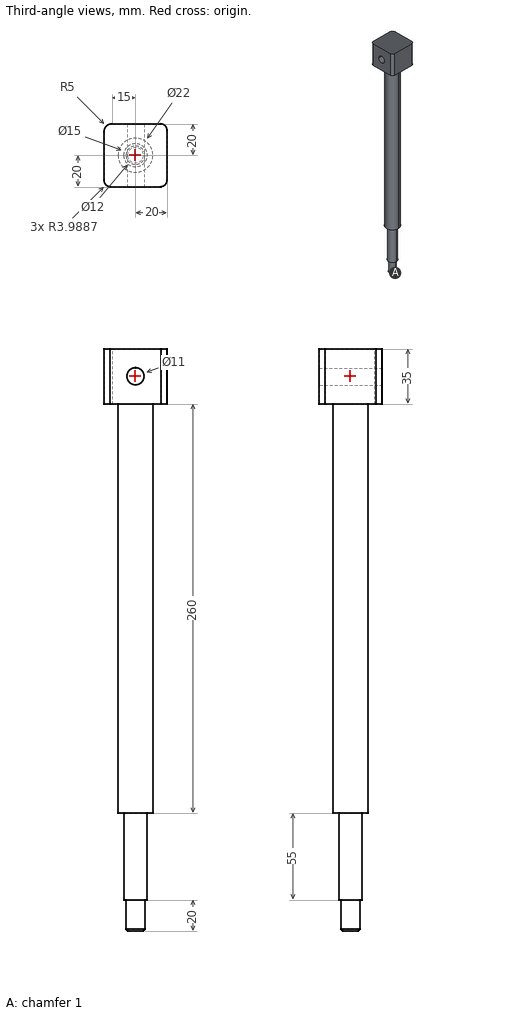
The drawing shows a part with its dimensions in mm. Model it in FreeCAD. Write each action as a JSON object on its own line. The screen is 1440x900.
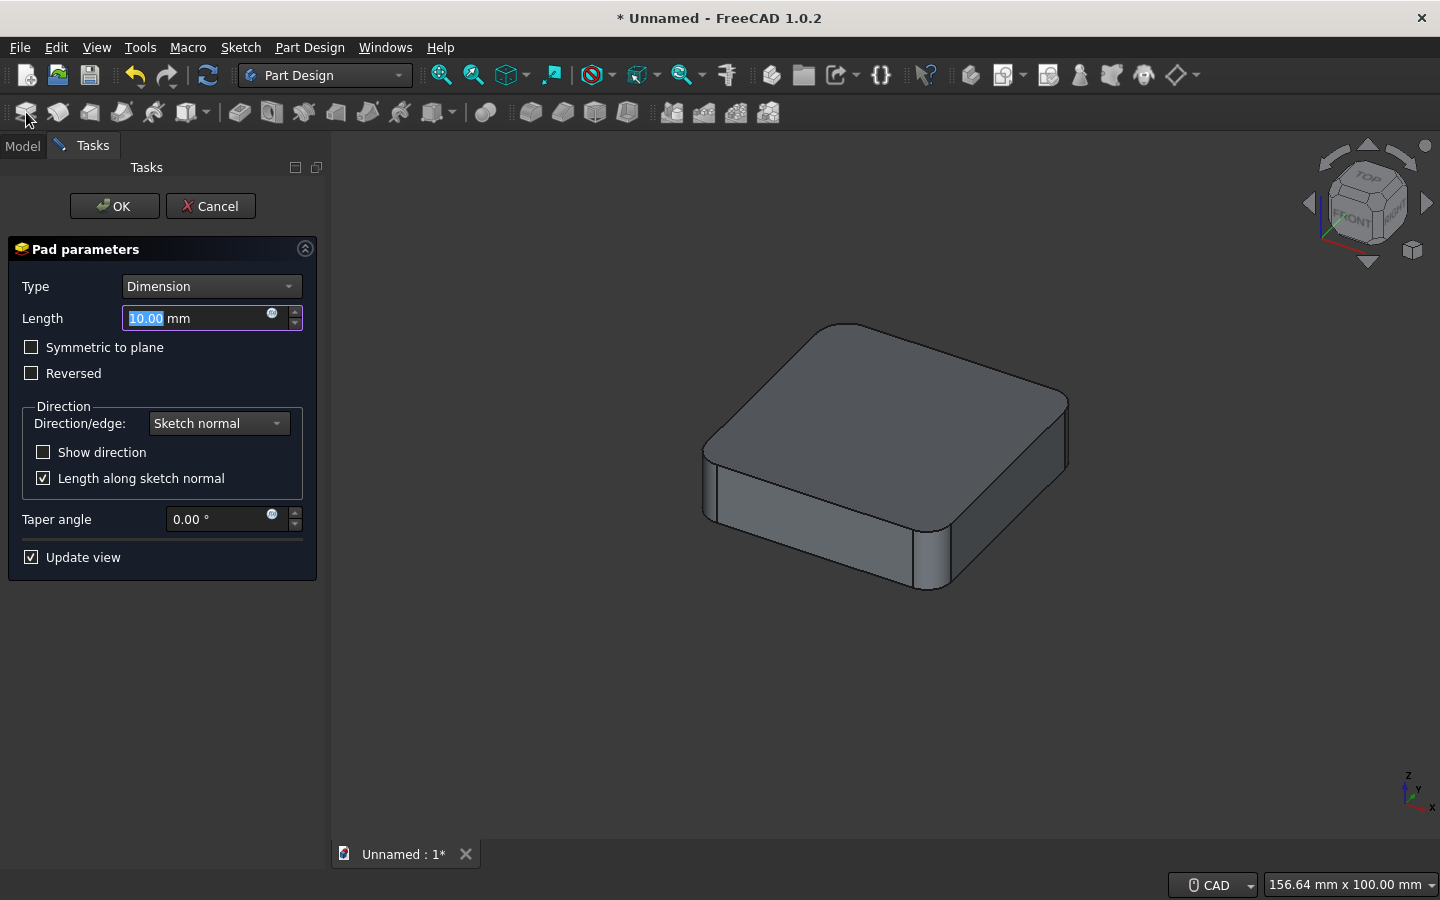
{"action": "type", "text": "35"}
{"action": "key", "text": "Tab"}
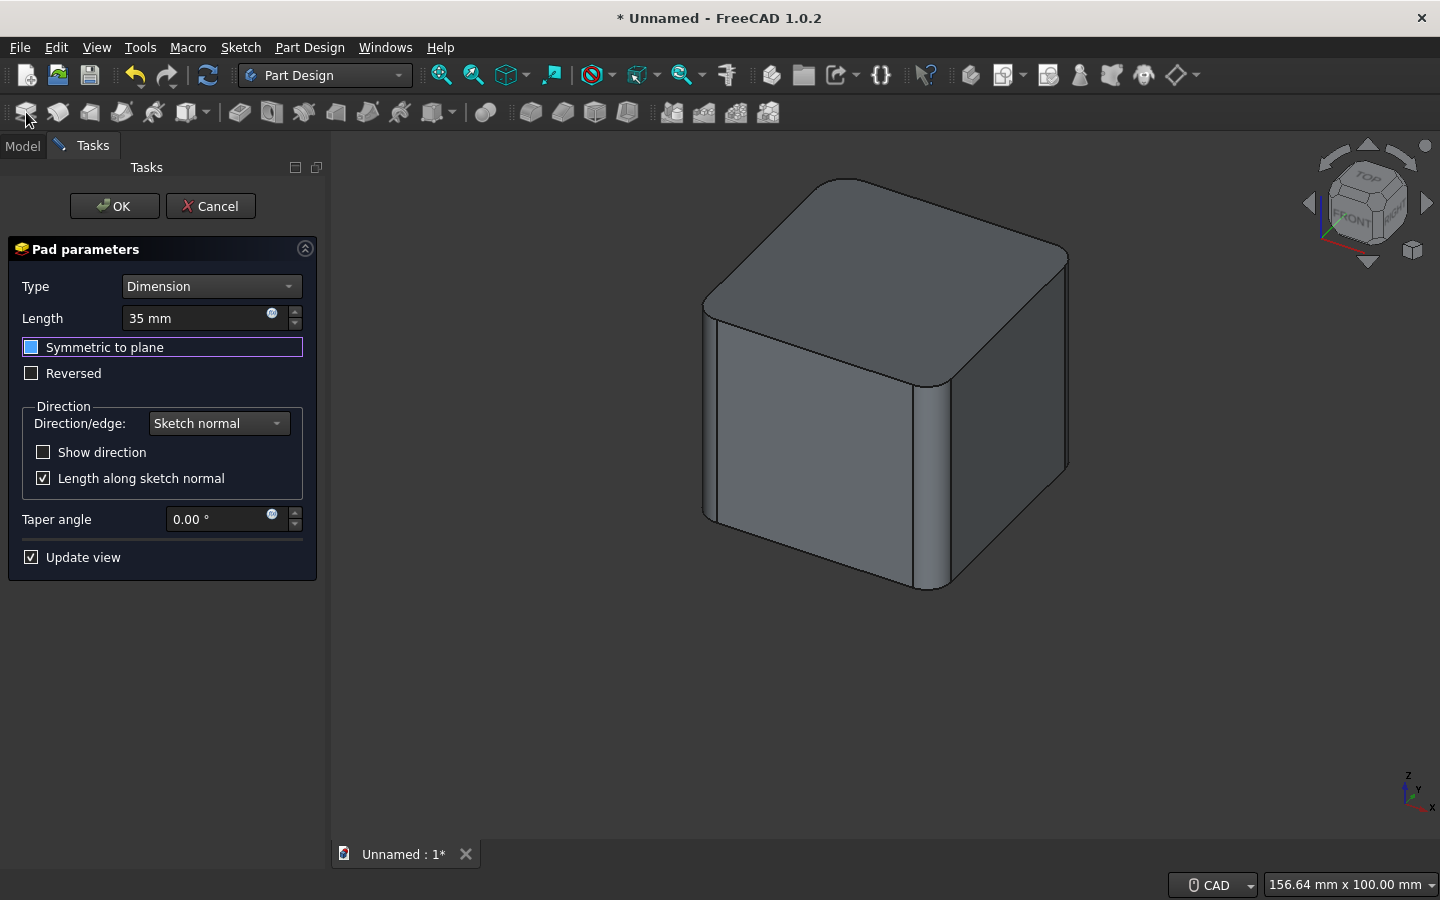
{"action": "left_click", "coordinate": [30, 347]}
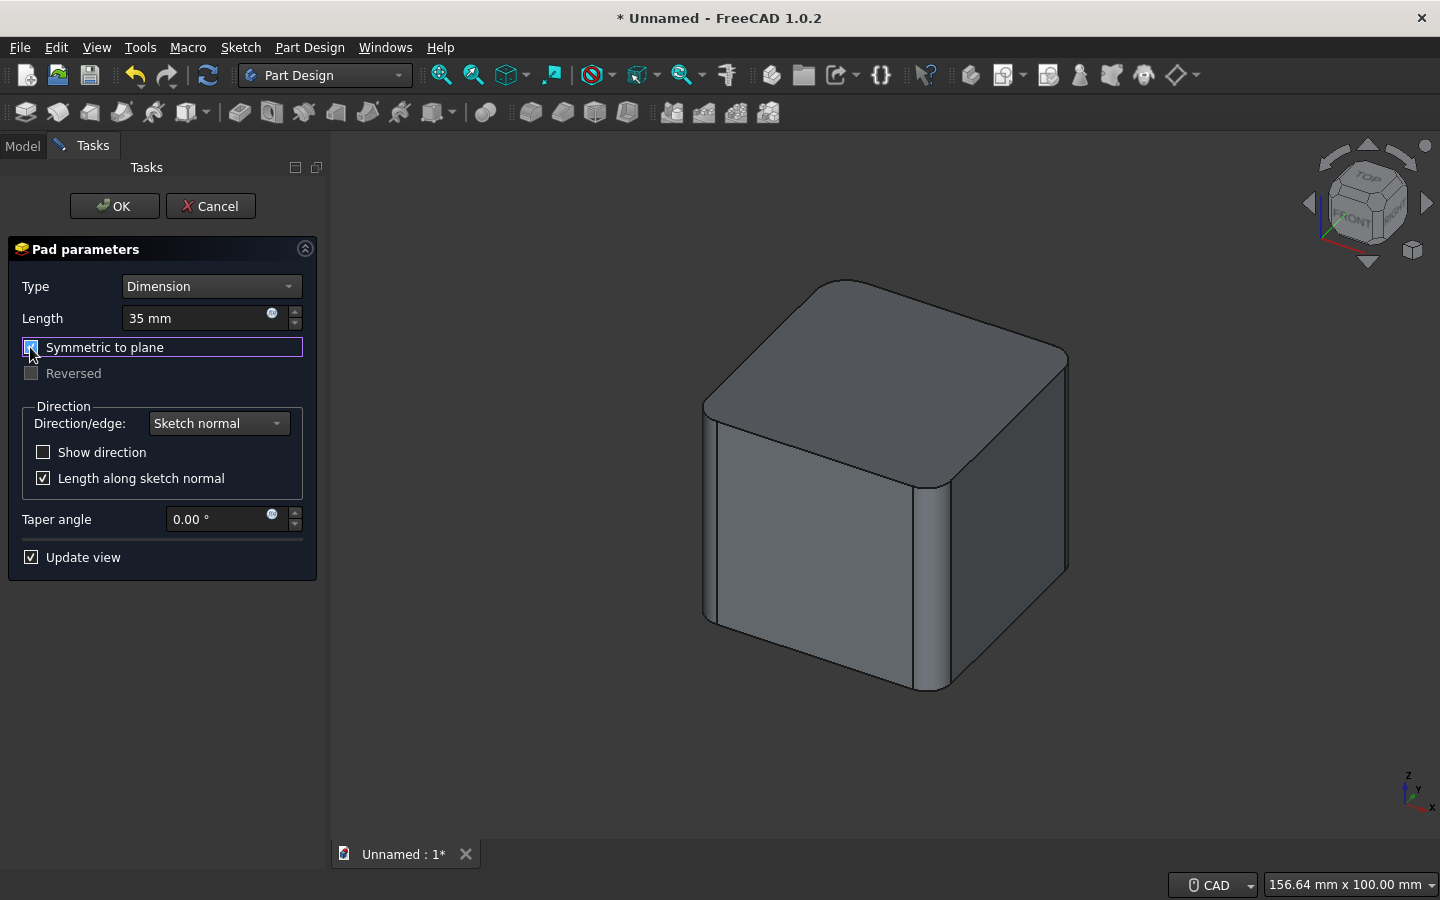
{"action": "left_click", "coordinate": [115, 206]}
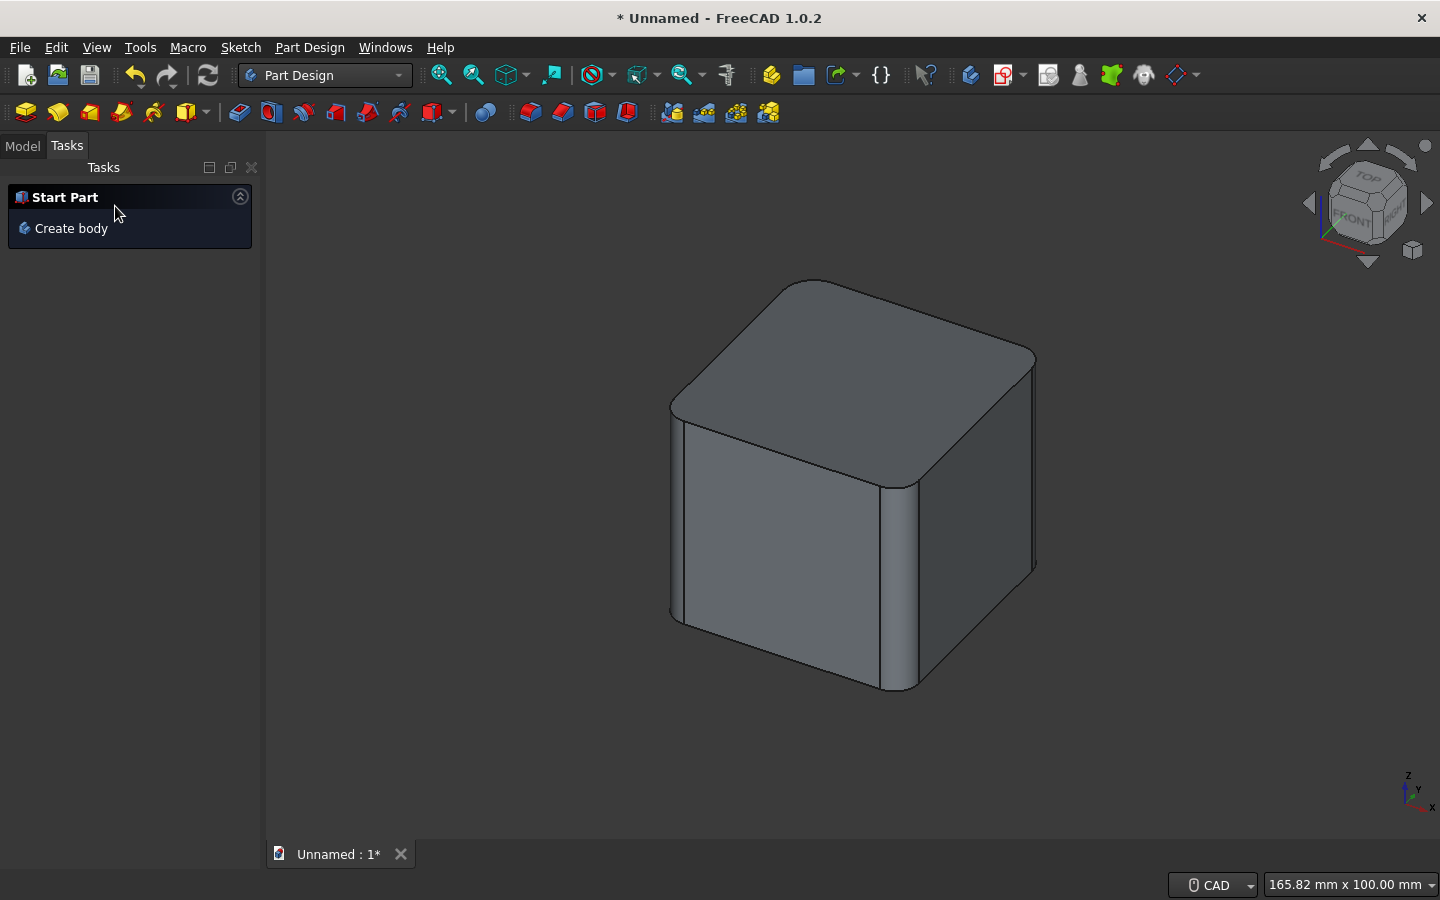
{"action": "key", "text": "4"}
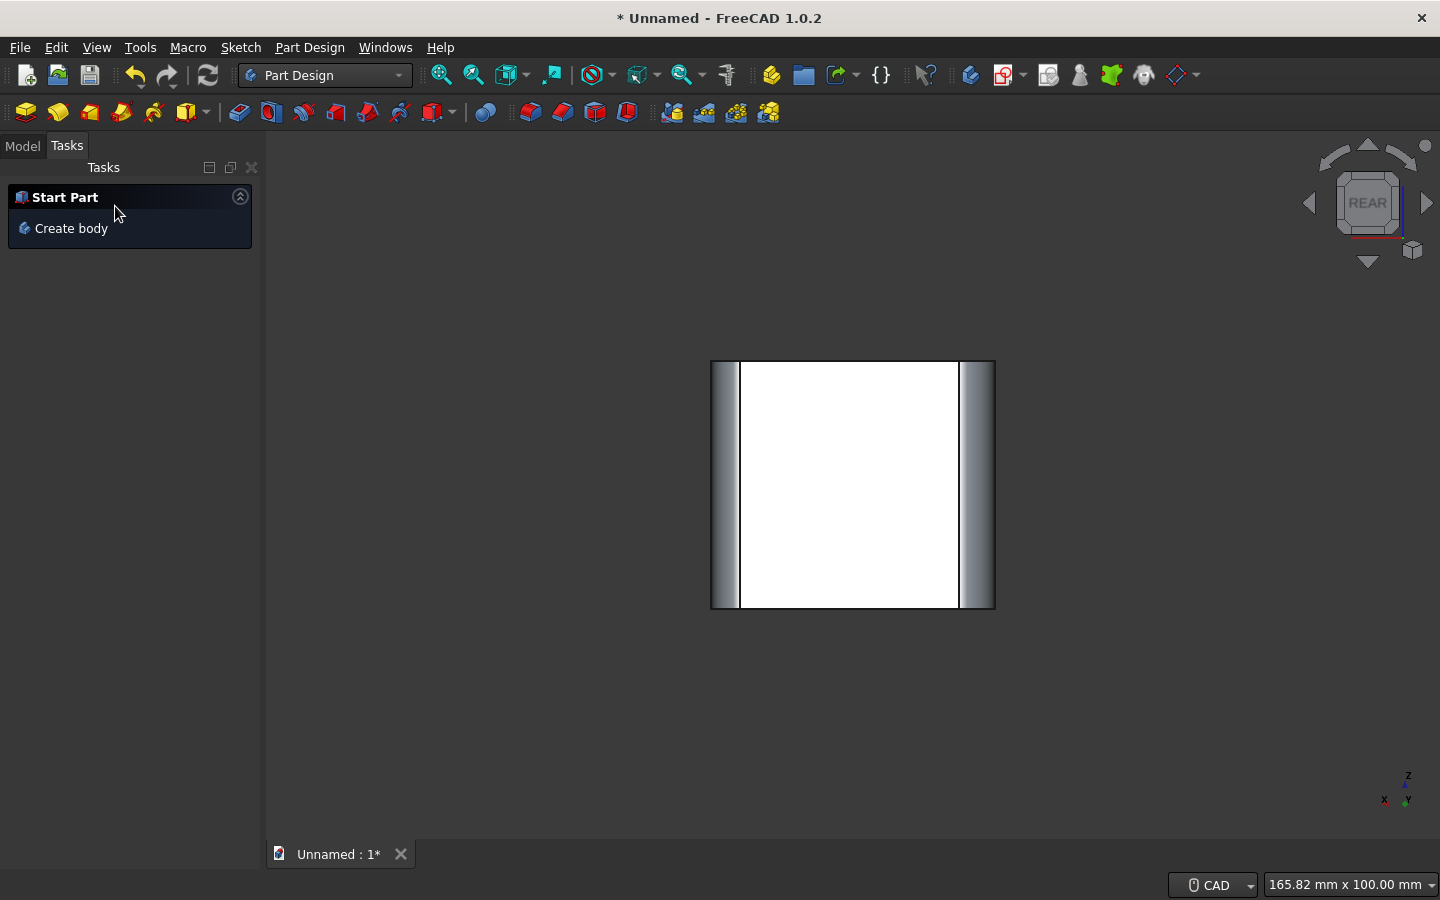
{"action": "key", "text": "v f"}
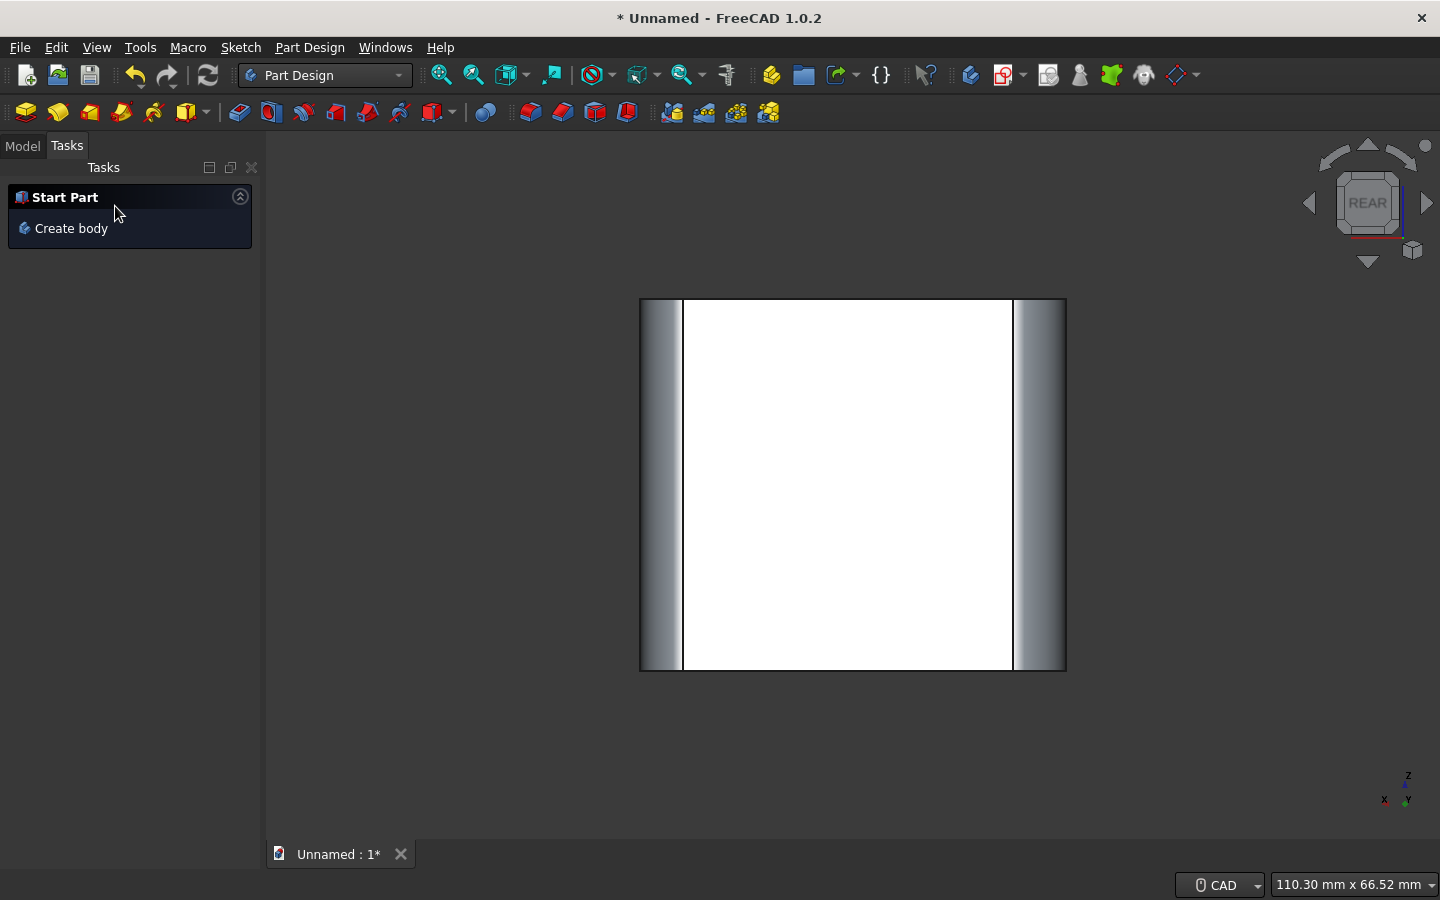
{"action": "left_click", "coordinate": [848, 484]}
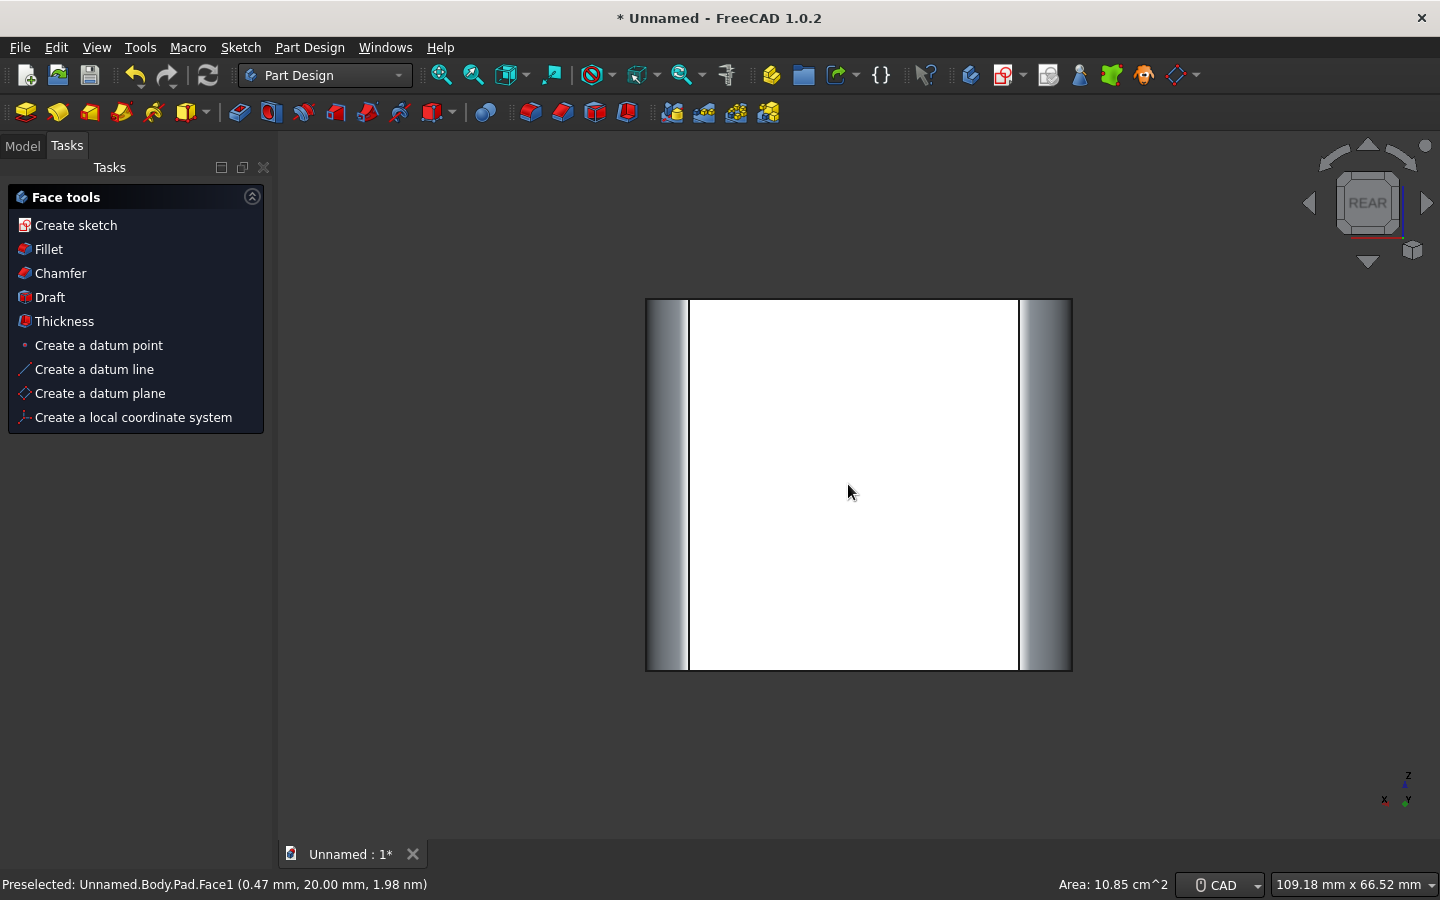
{"action": "left_click", "coordinate": [1004, 76]}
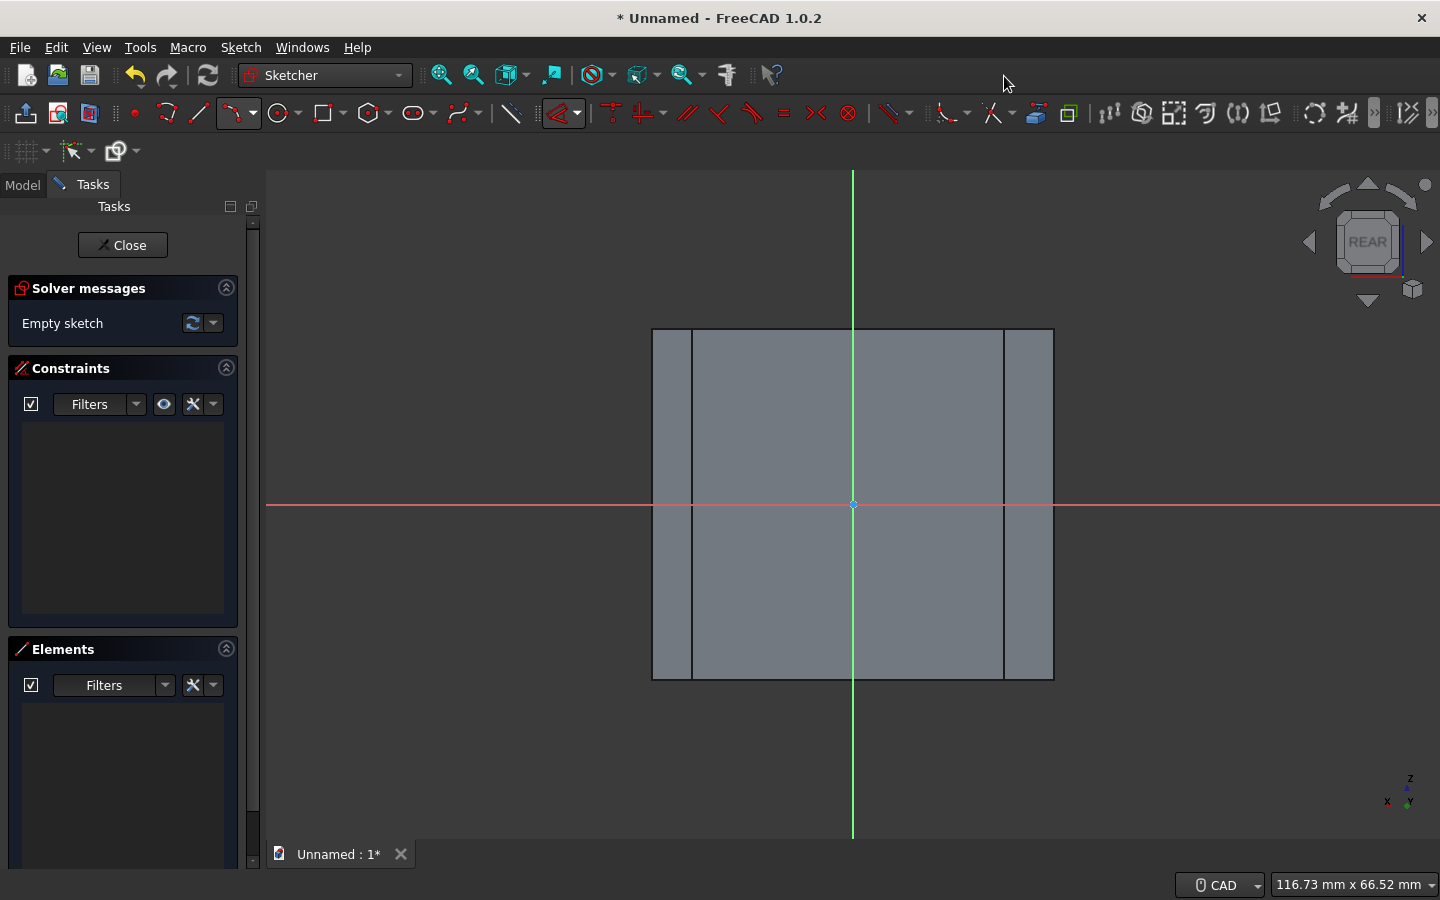
{"action": "scroll", "coordinate": [875, 504], "scroll_direction": "up", "scroll_amount": 7}